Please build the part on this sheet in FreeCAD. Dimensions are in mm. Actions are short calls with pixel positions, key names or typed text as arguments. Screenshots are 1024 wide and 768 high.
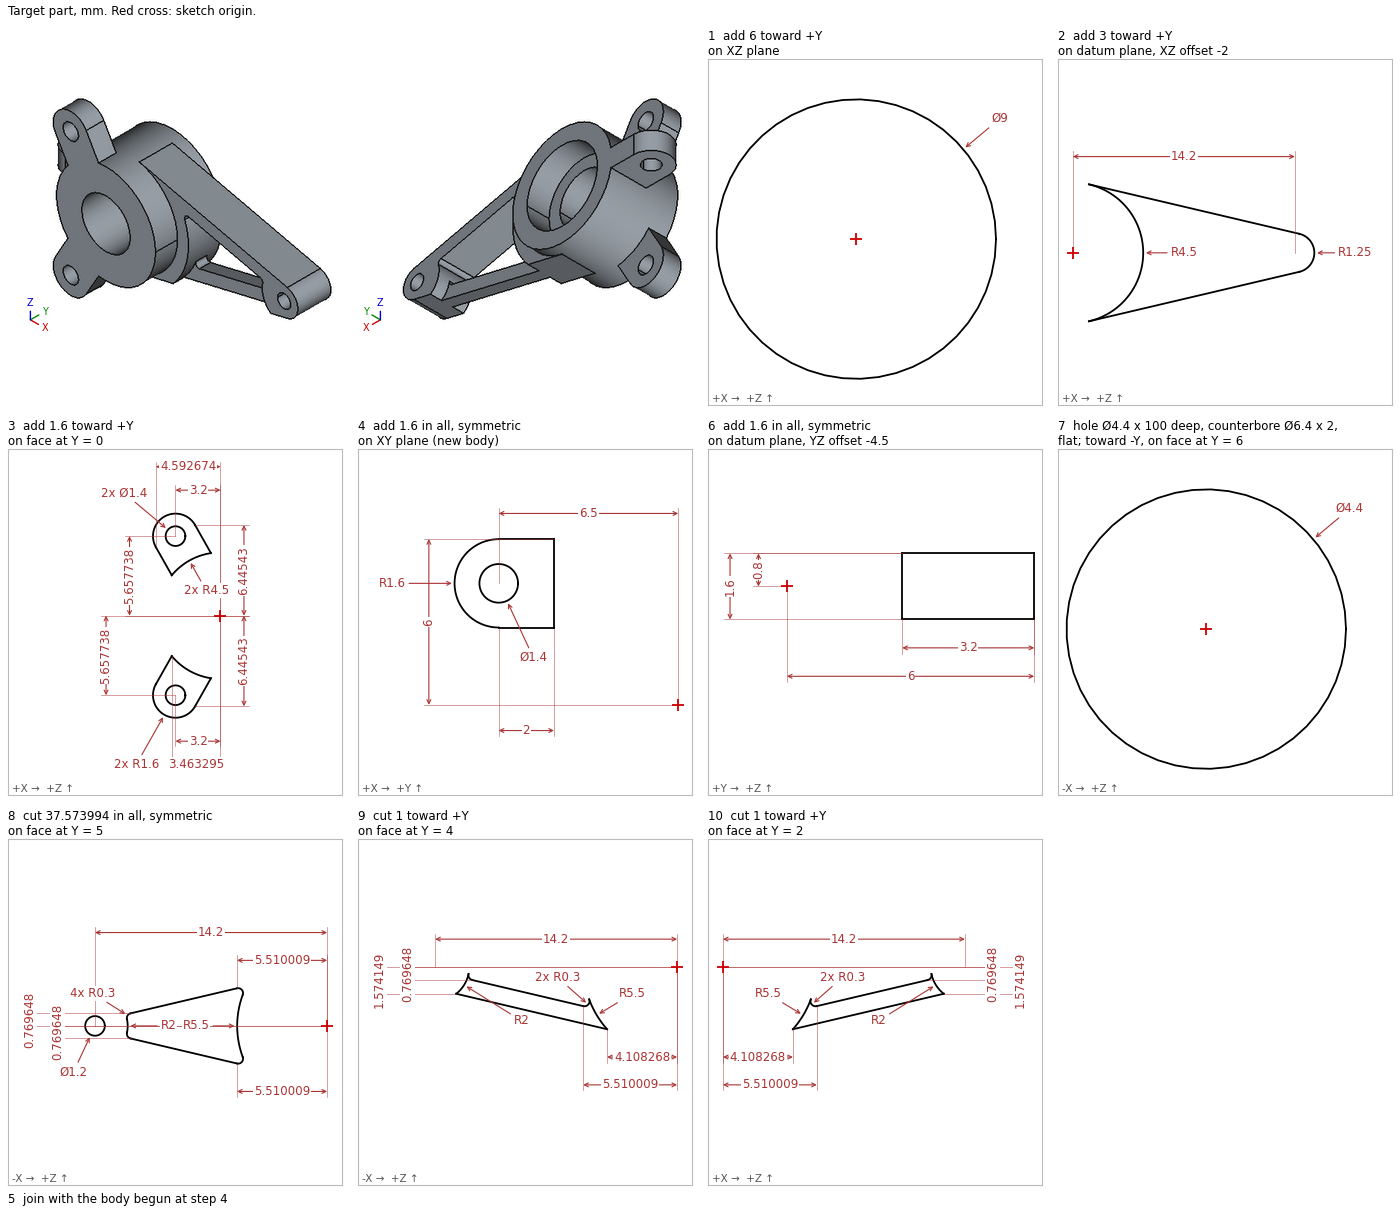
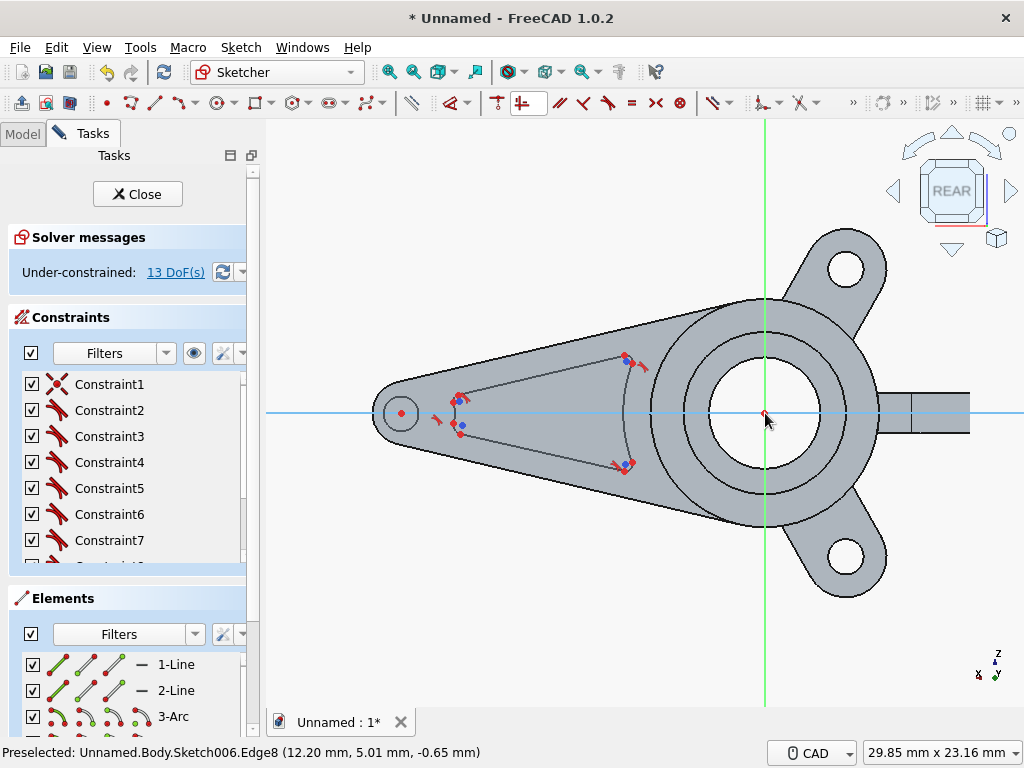
scroll(629, 471, up, 6)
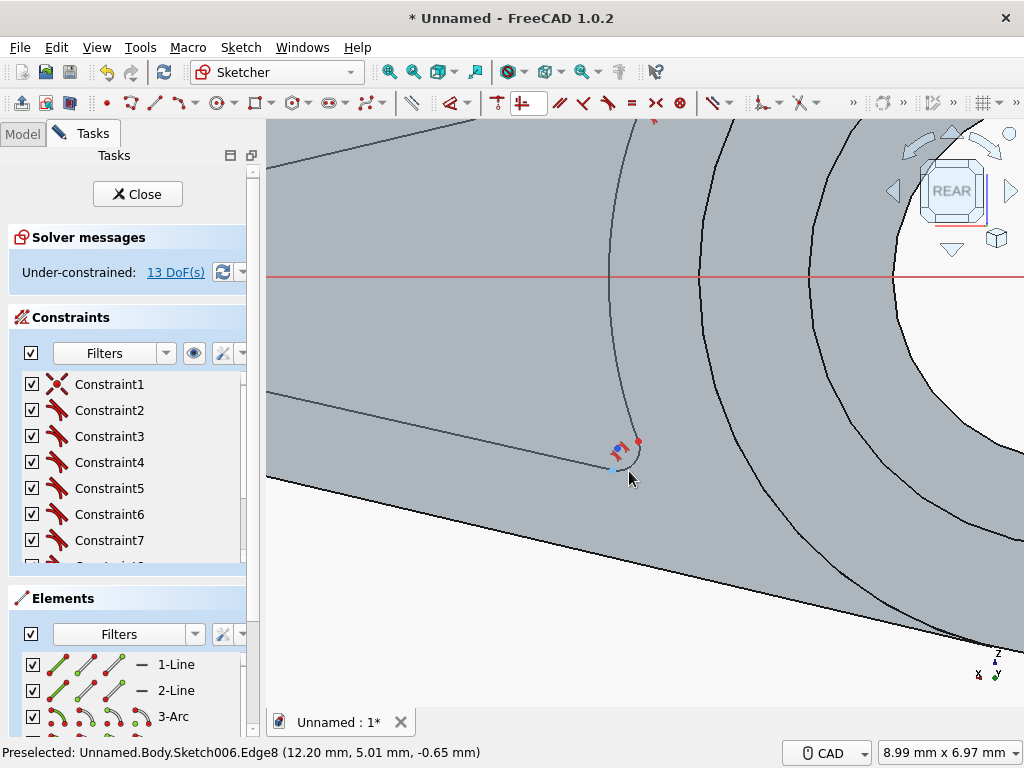
click(627, 469)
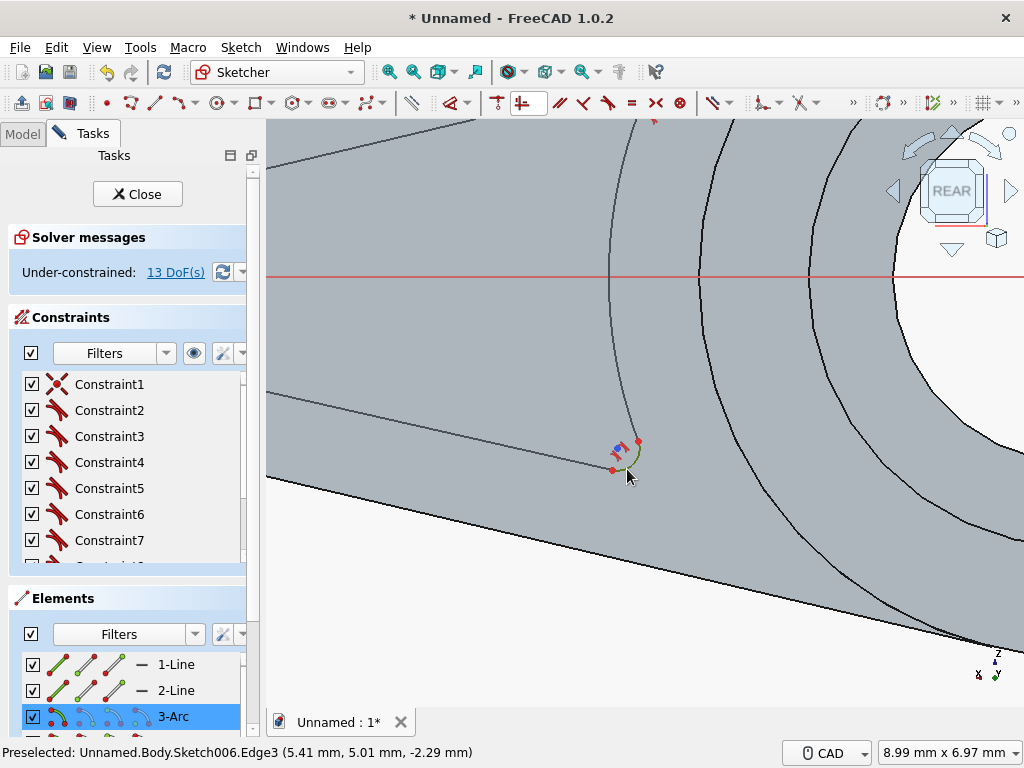
scroll(629, 471, down, 6)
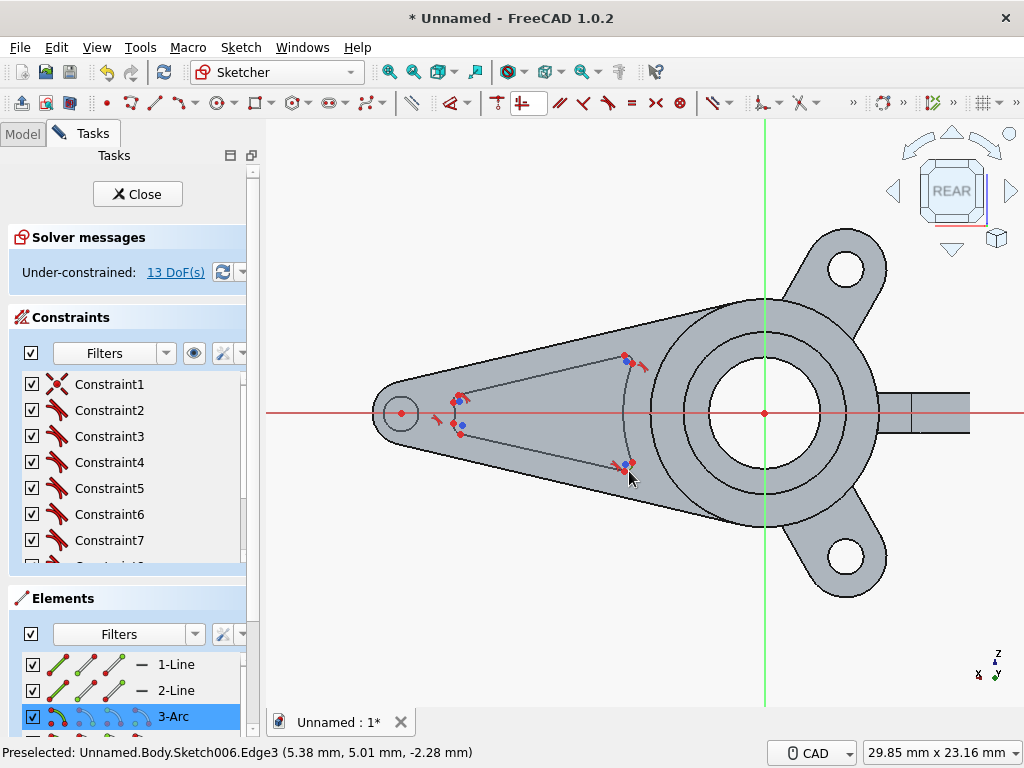
scroll(632, 360, up, 7)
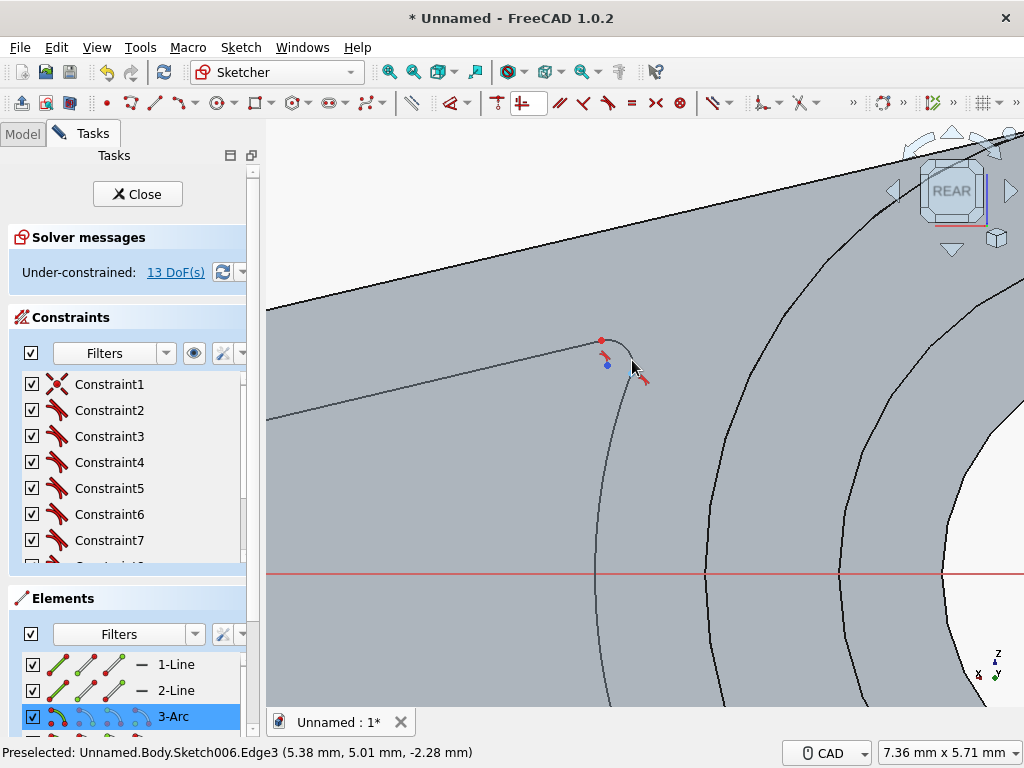
click(632, 358)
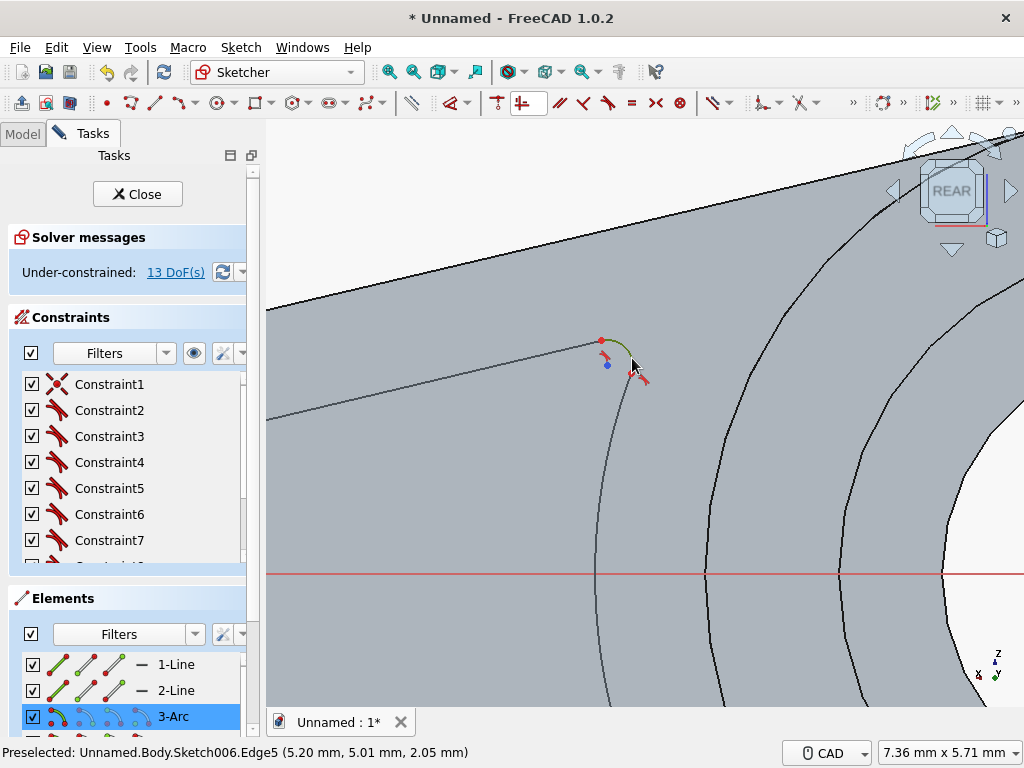
scroll(632, 360, down, 7)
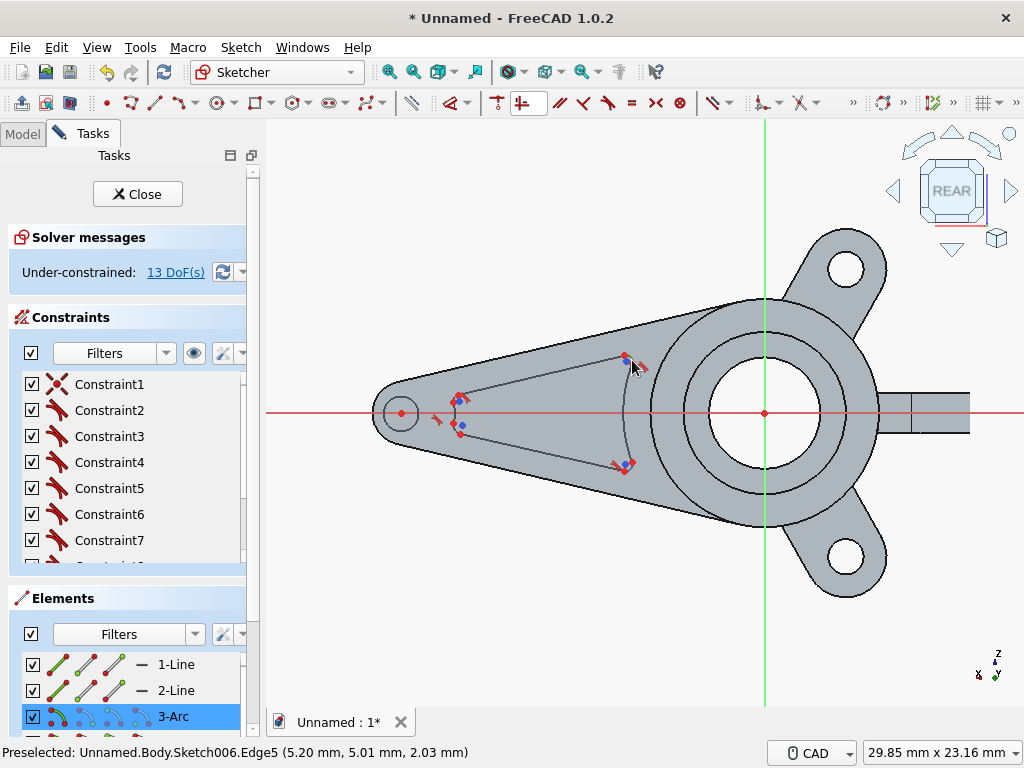
scroll(456, 396, up, 8)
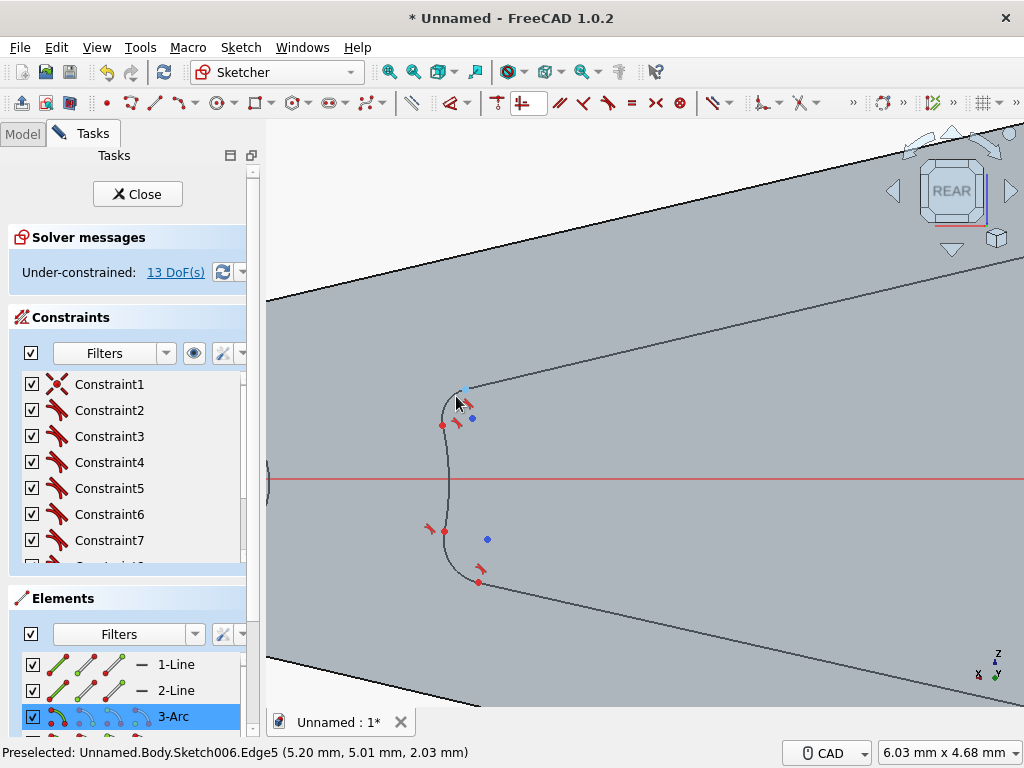
click(453, 396)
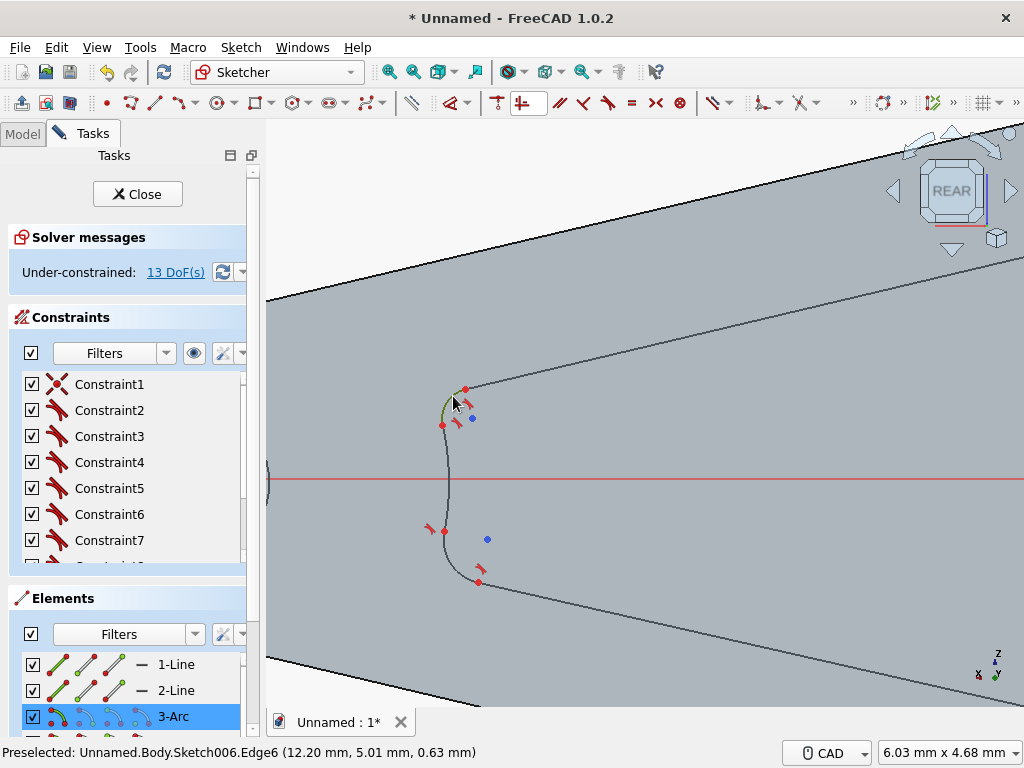
click(445, 552)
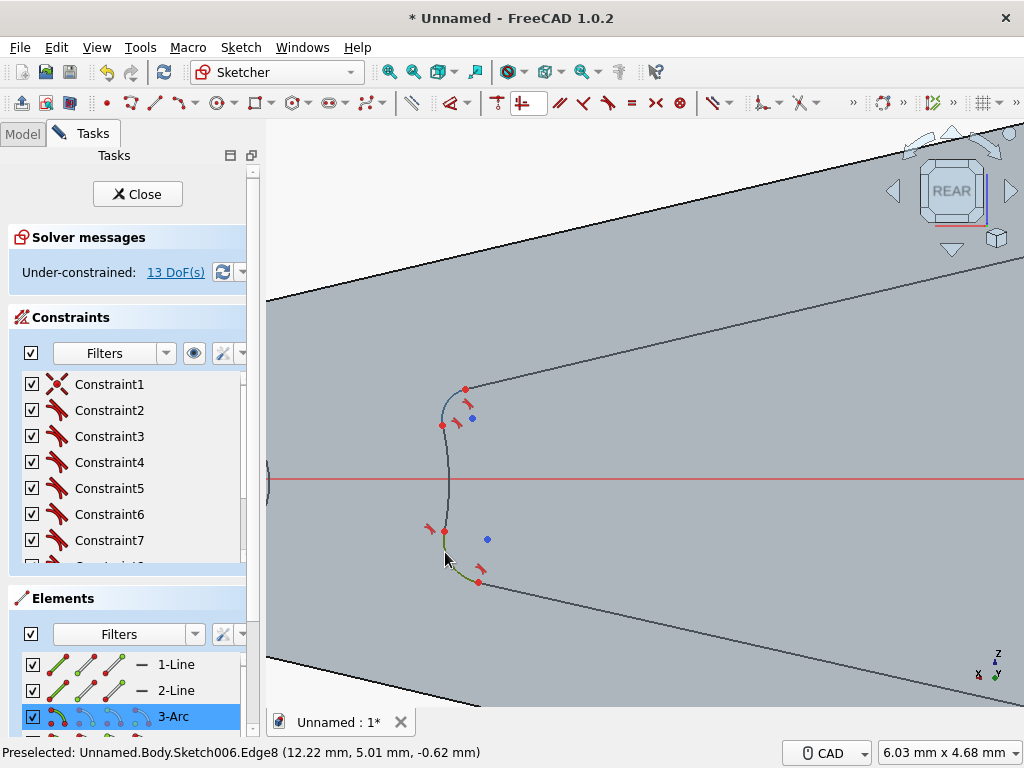
key(e)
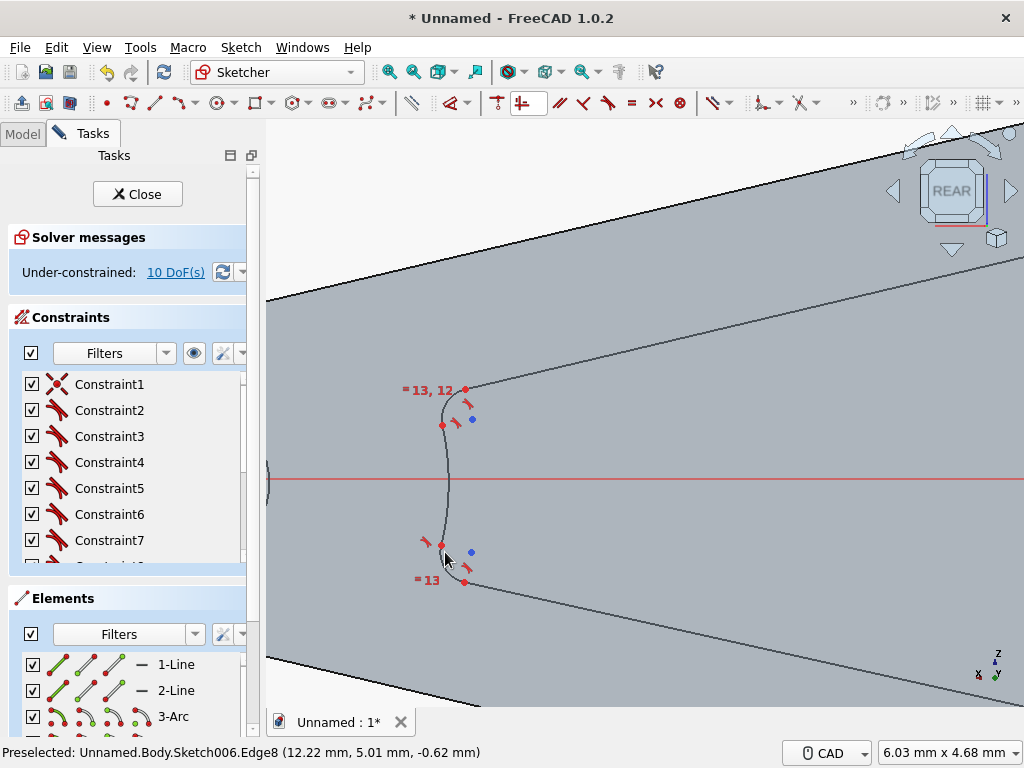
scroll(456, 396, down, 8)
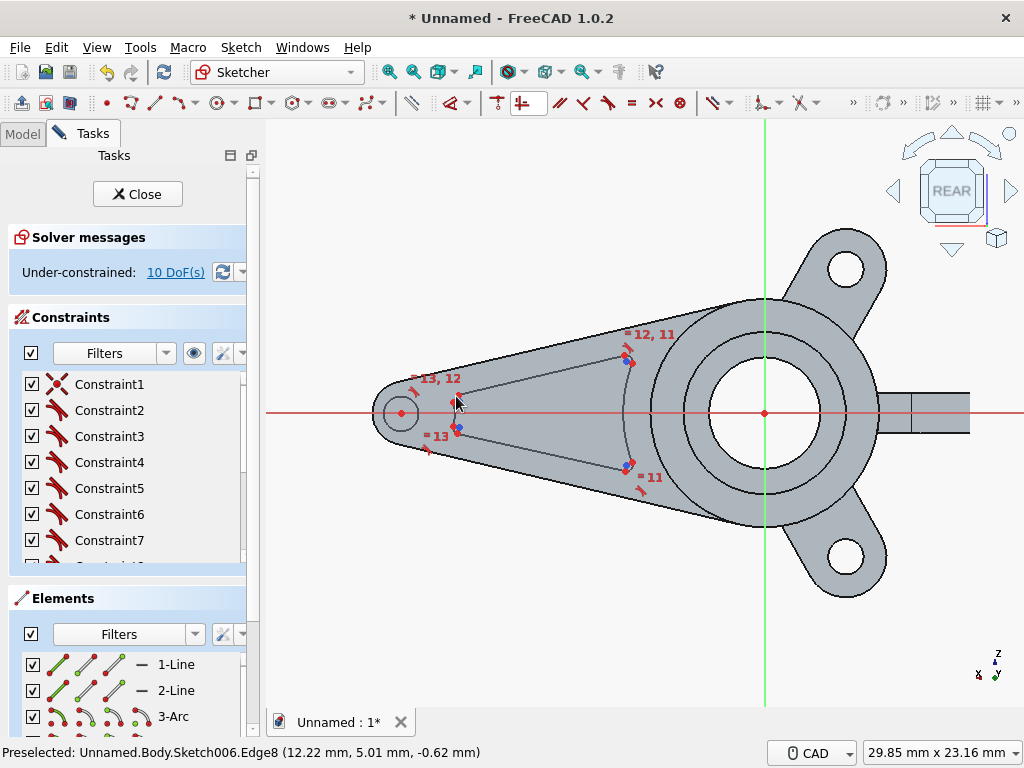
click(401, 414)